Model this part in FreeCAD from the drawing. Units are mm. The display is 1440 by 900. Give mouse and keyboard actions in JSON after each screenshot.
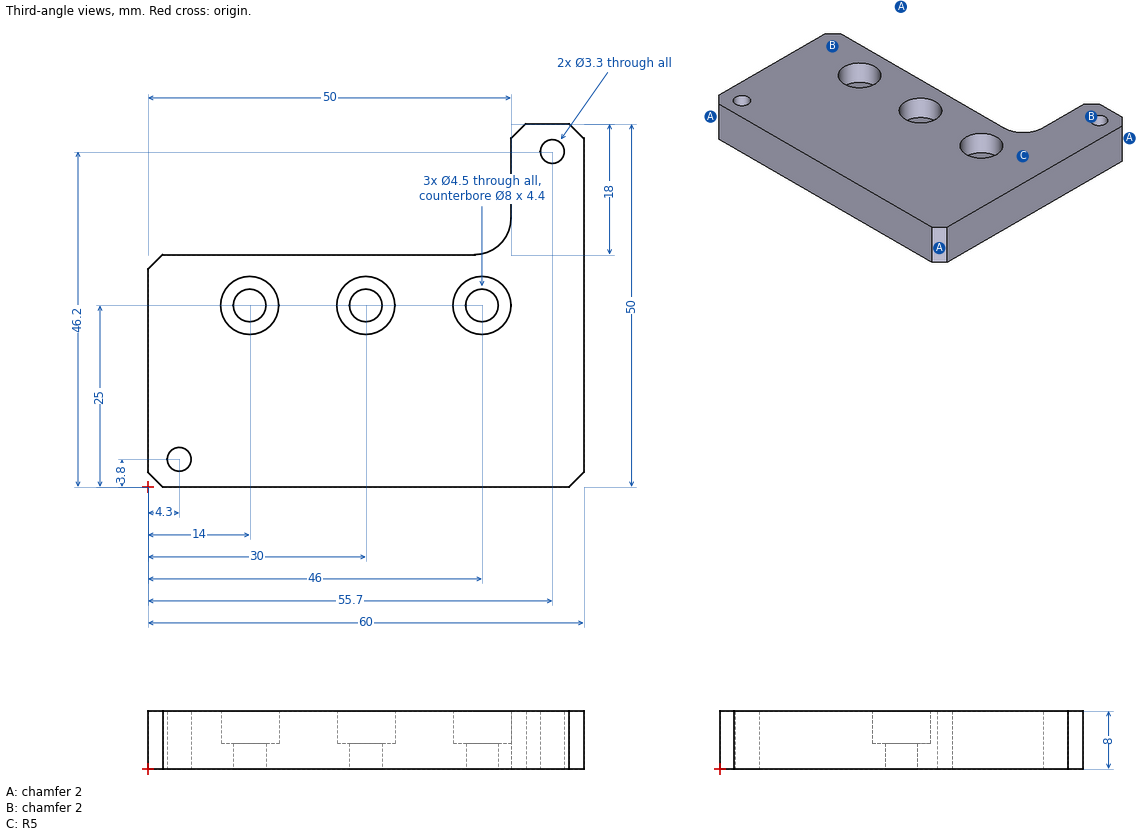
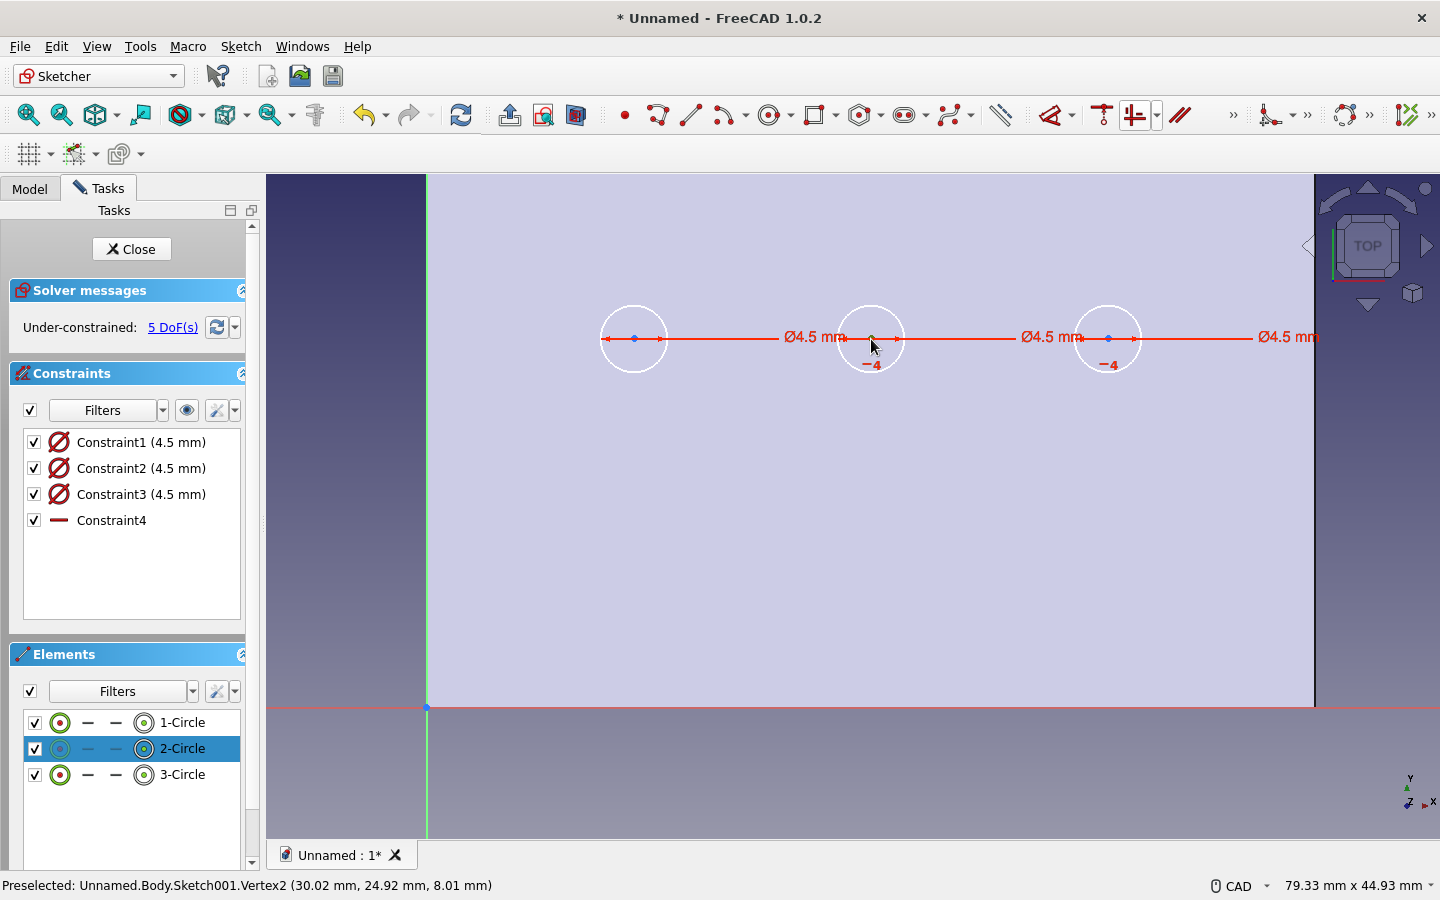
{"action": "left_click", "coordinate": [634, 339]}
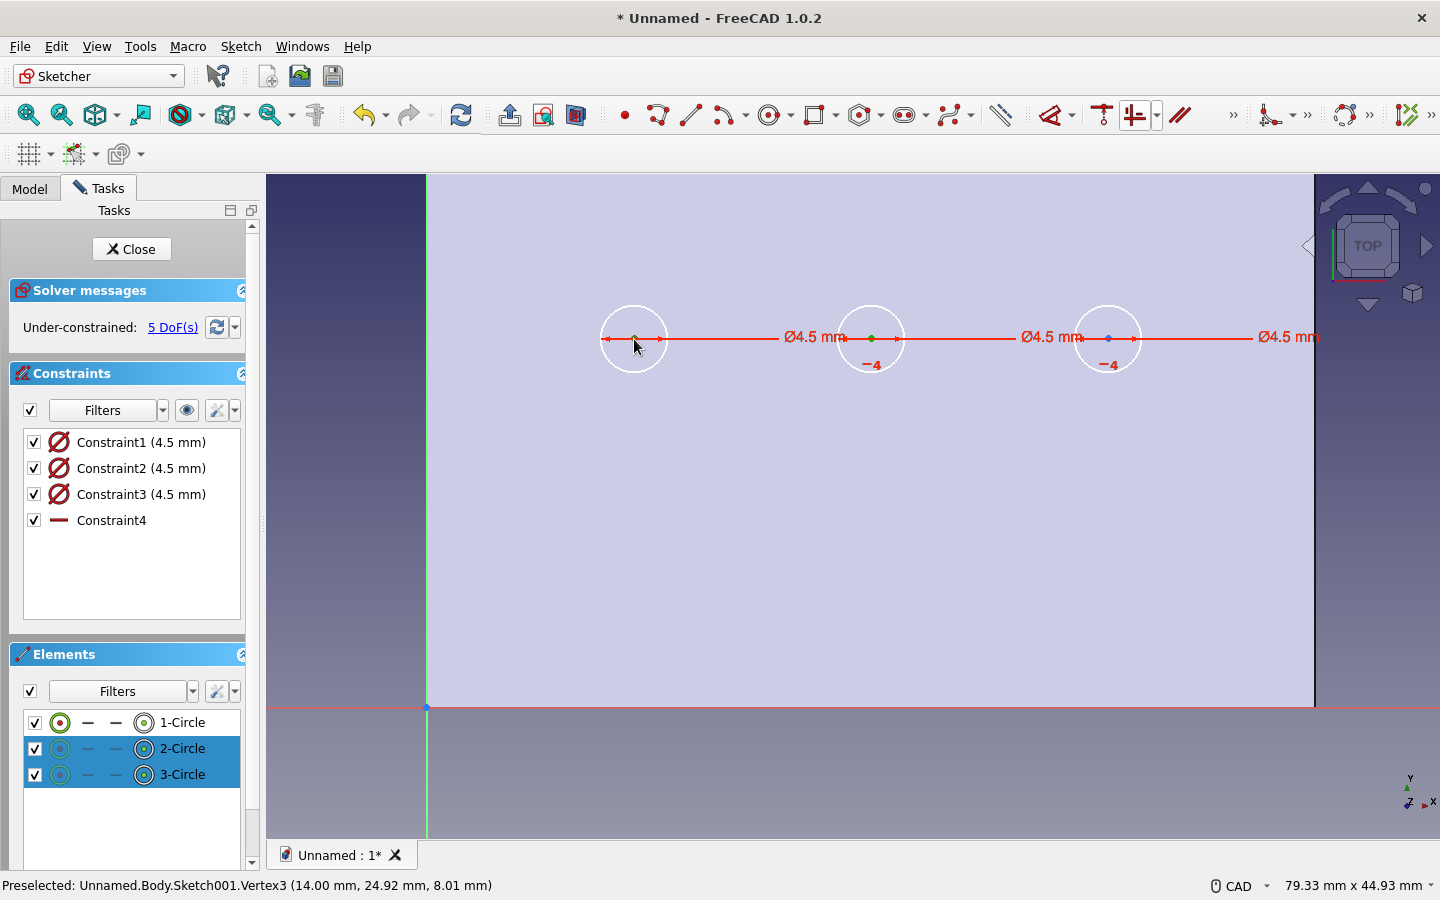
{"action": "key", "text": "h"}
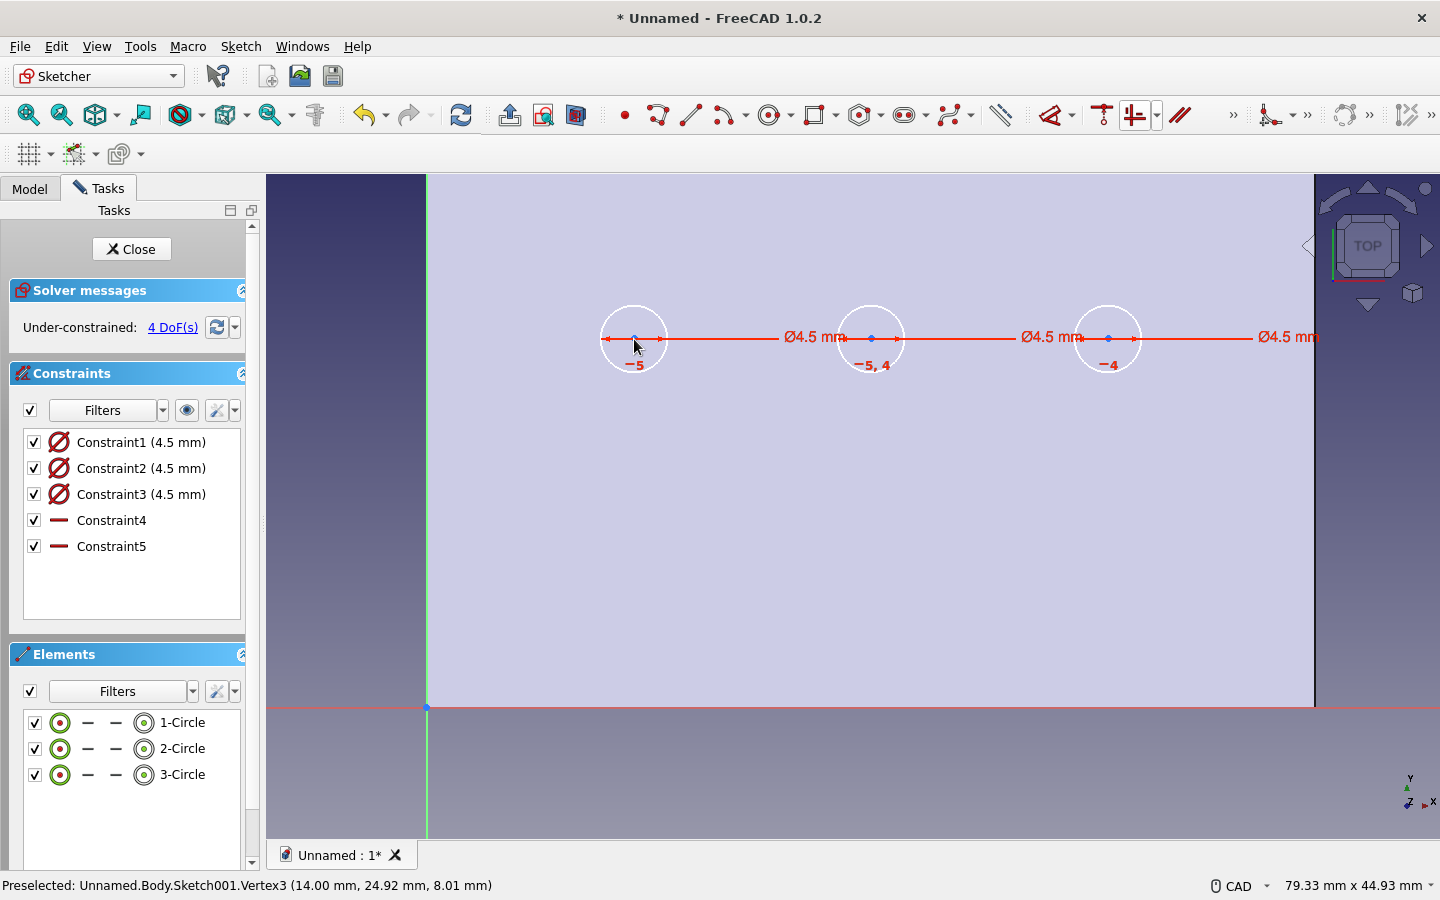
{"action": "left_click", "coordinate": [1050, 116]}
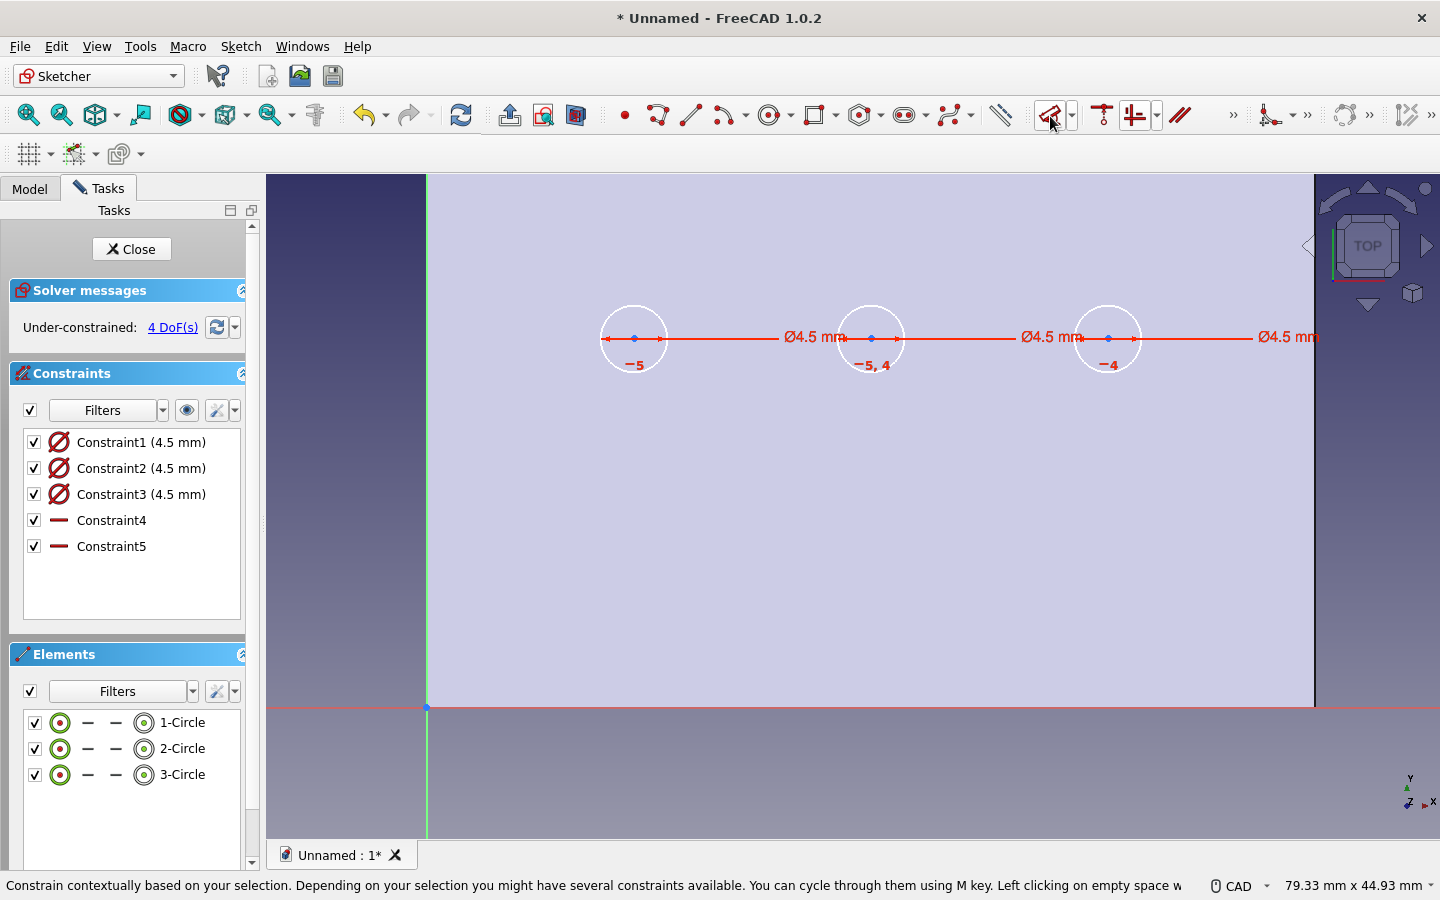
{"action": "left_click", "coordinate": [1108, 339]}
{"action": "left_click", "coordinate": [767, 742]}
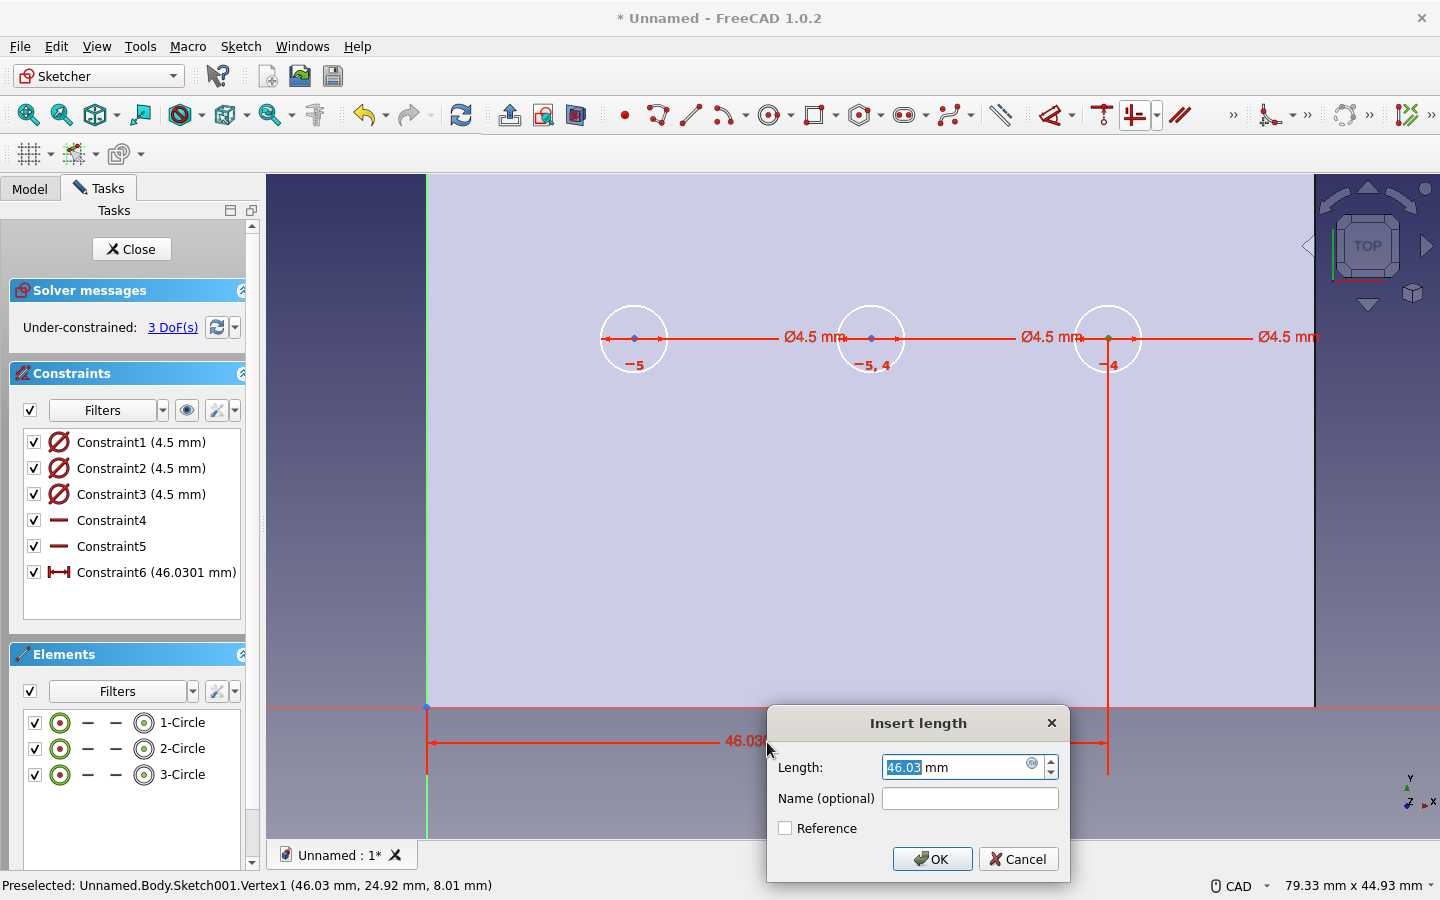
{"action": "type", "text": "46"}
{"action": "key", "text": "Return"}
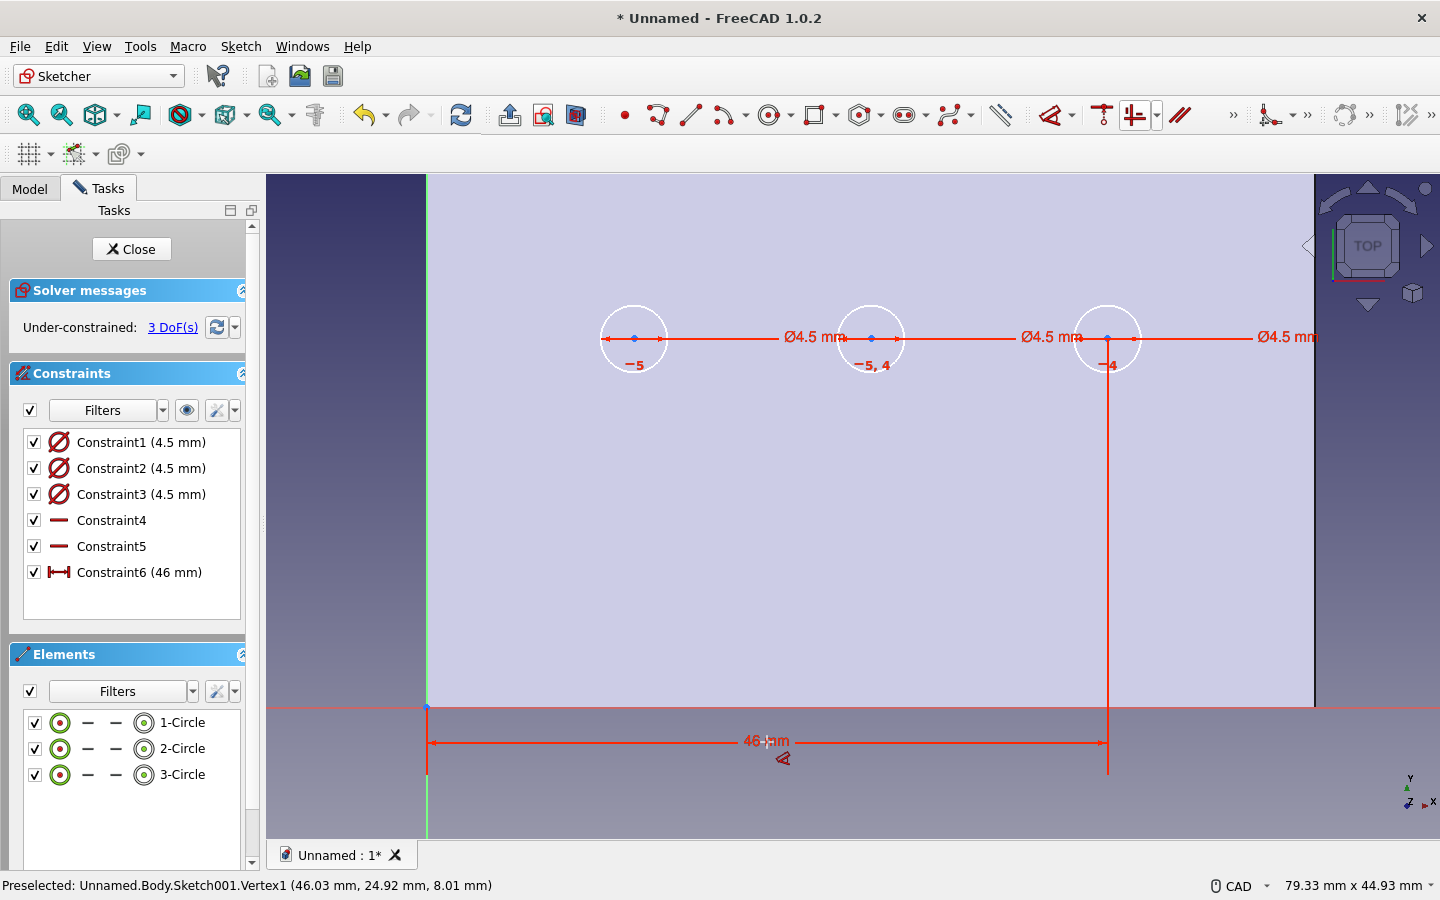
{"action": "left_click", "coordinate": [1108, 339]}
{"action": "left_click", "coordinate": [393, 523]}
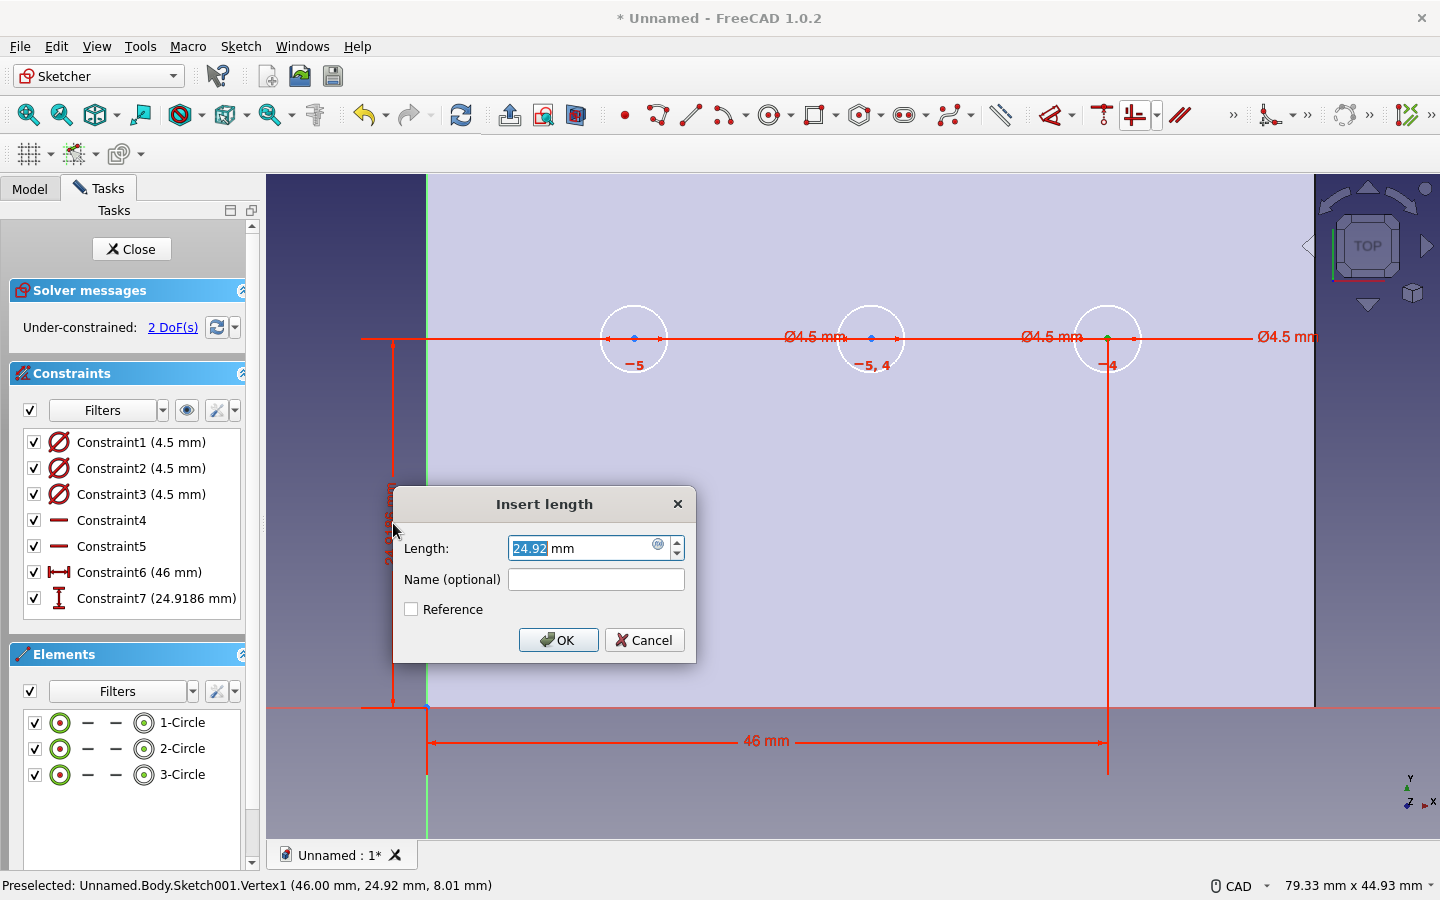
{"action": "type", "text": "25"}
{"action": "key", "text": "Return"}